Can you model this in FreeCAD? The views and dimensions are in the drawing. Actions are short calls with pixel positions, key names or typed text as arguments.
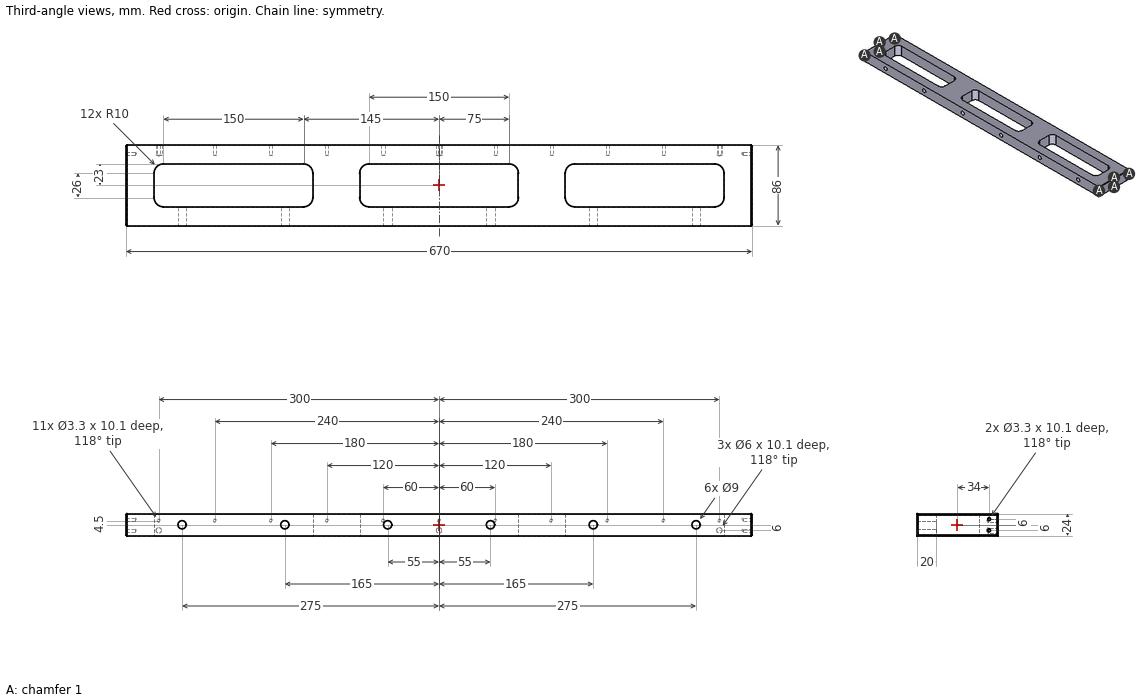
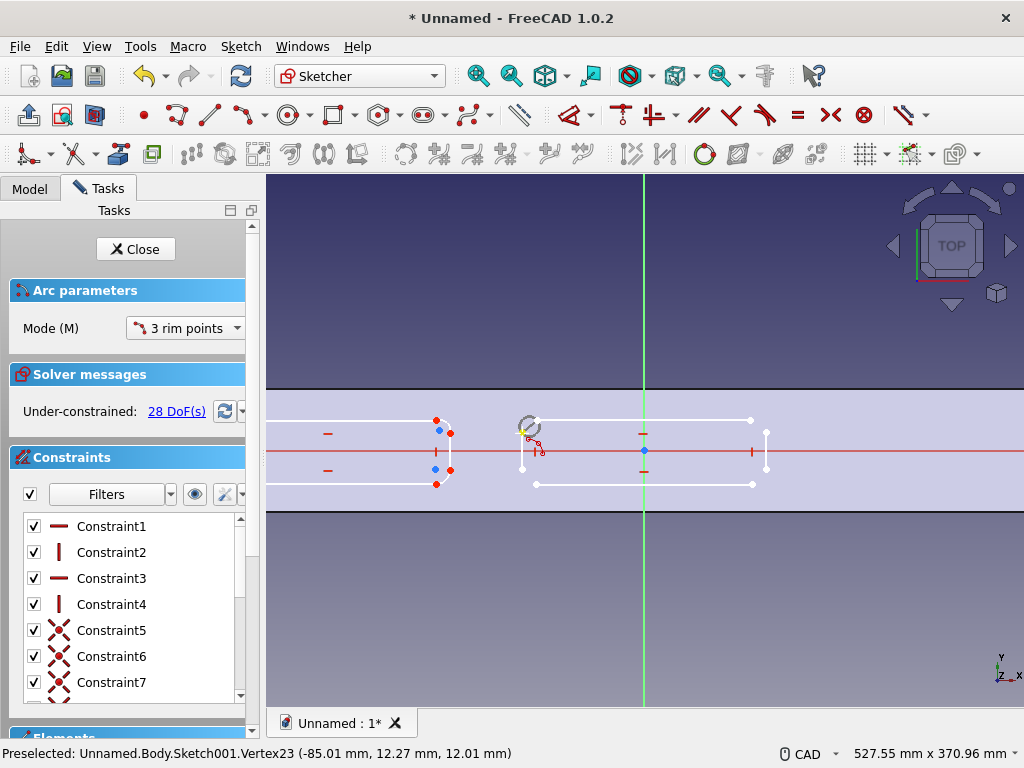
scroll(526, 422, up, 7)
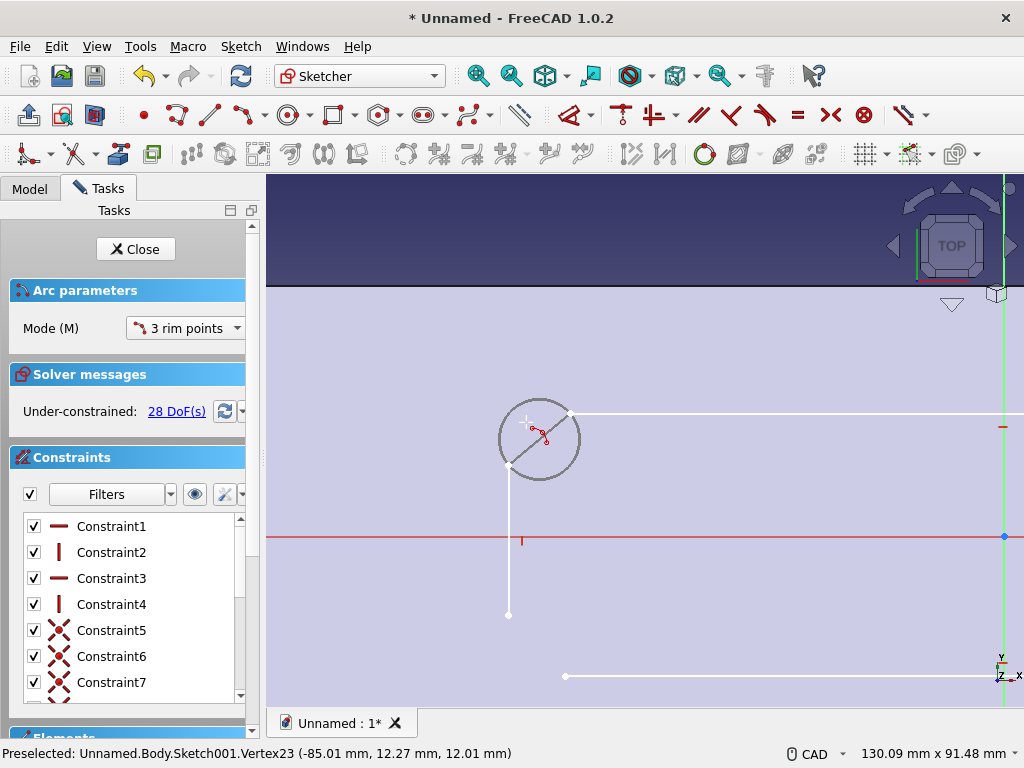
click(526, 420)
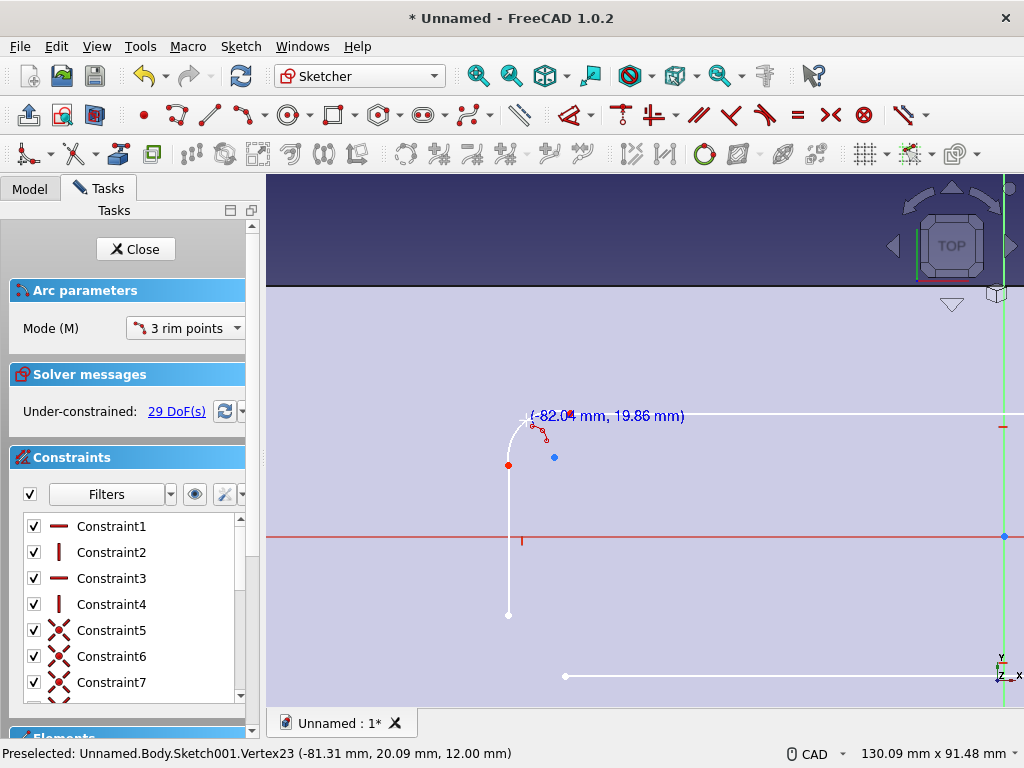
scroll(523, 429, down, 11)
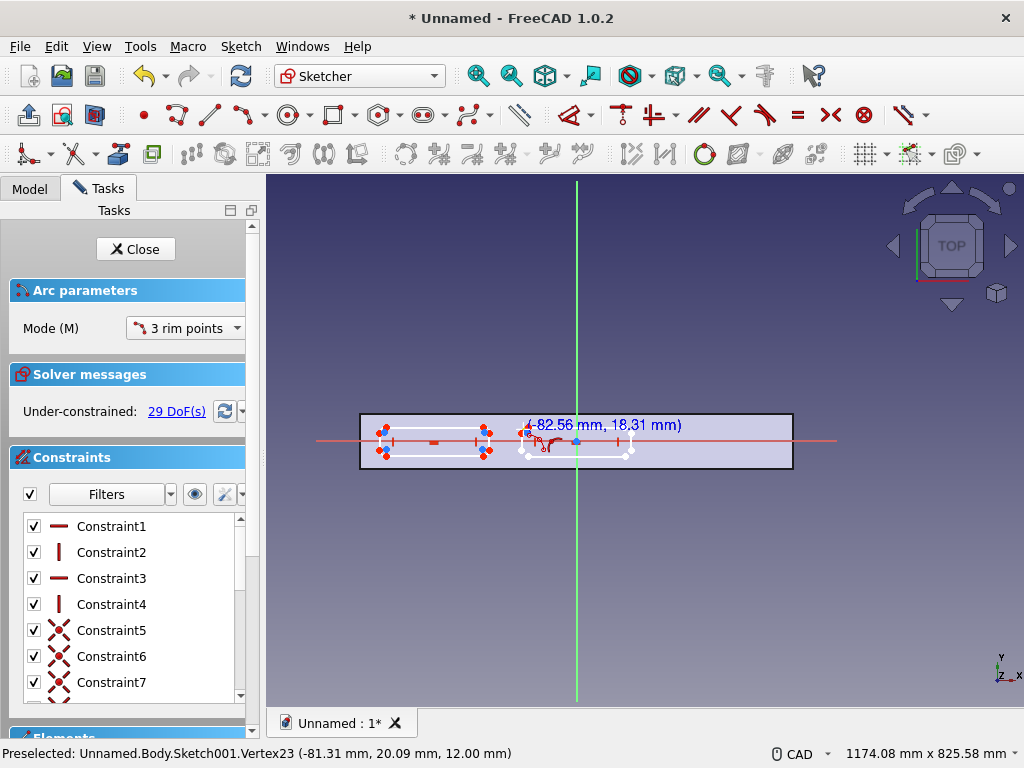
scroll(522, 450, up, 4)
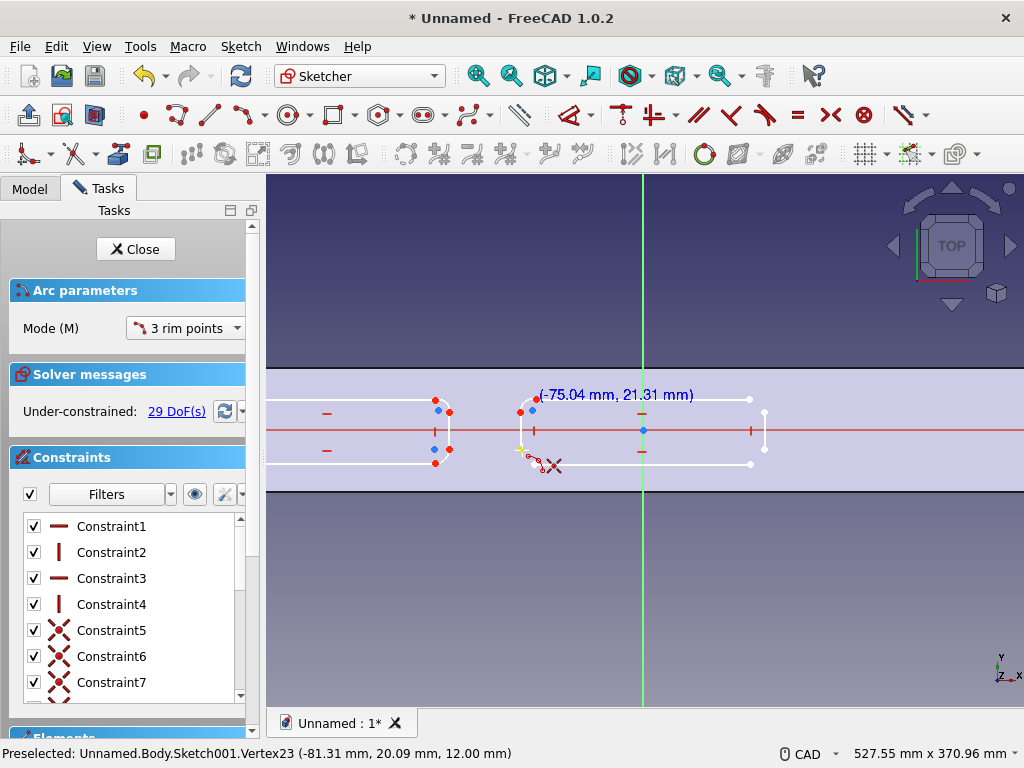
click(521, 449)
click(535, 464)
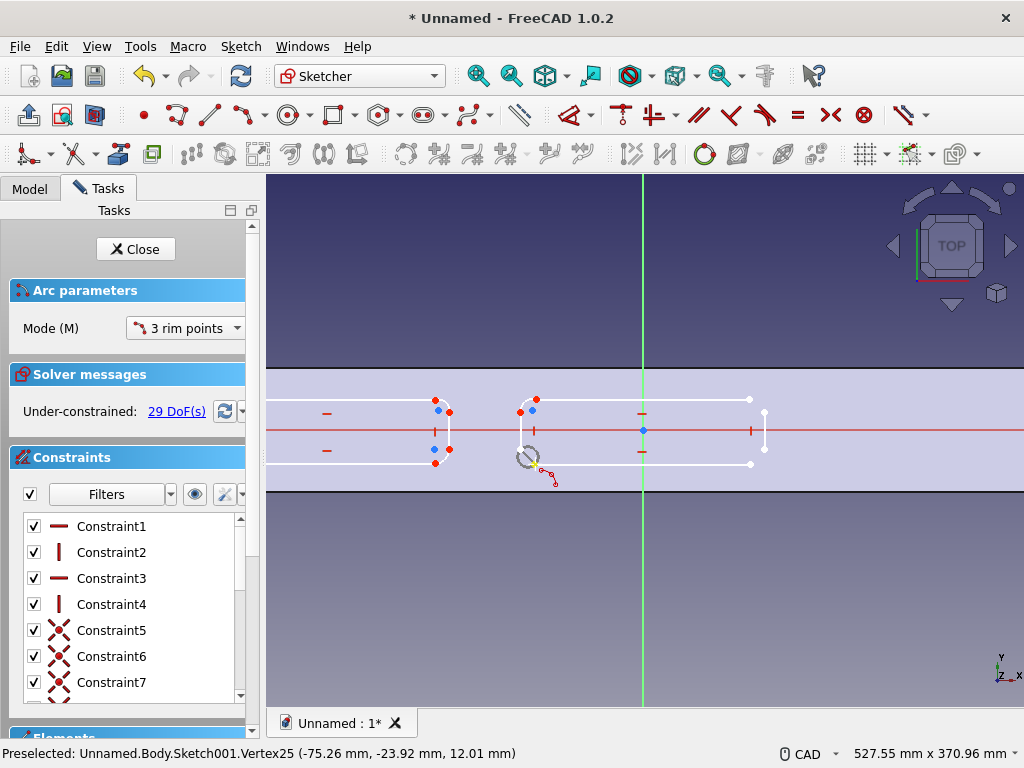
scroll(525, 459, up, 7)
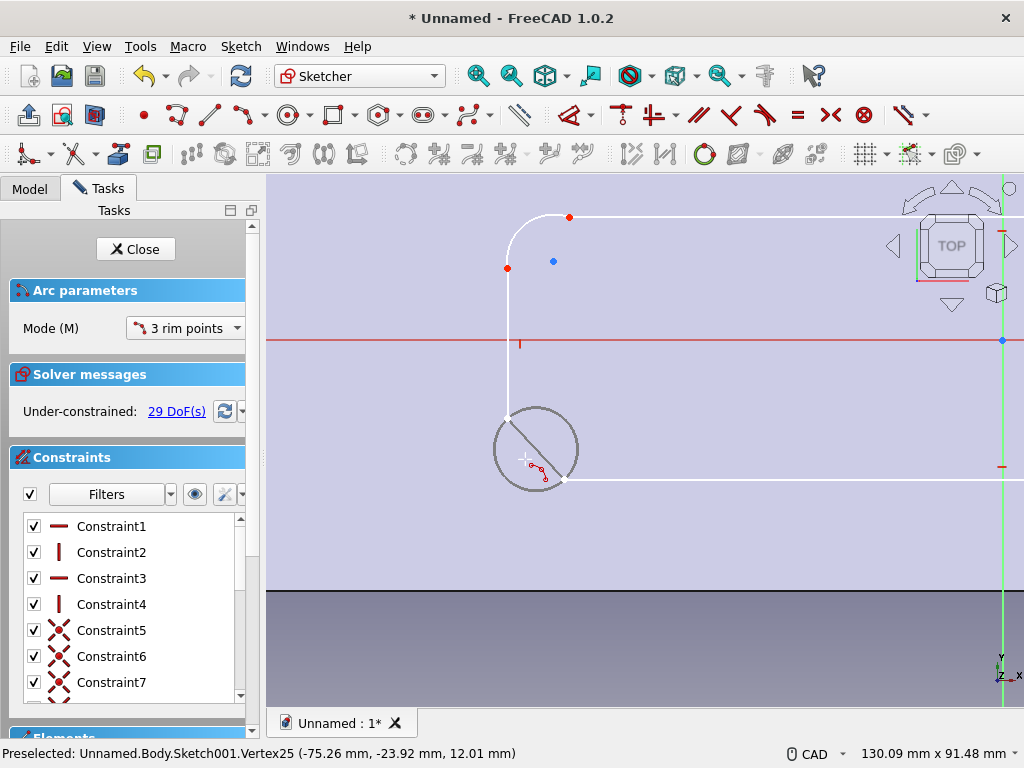
click(525, 457)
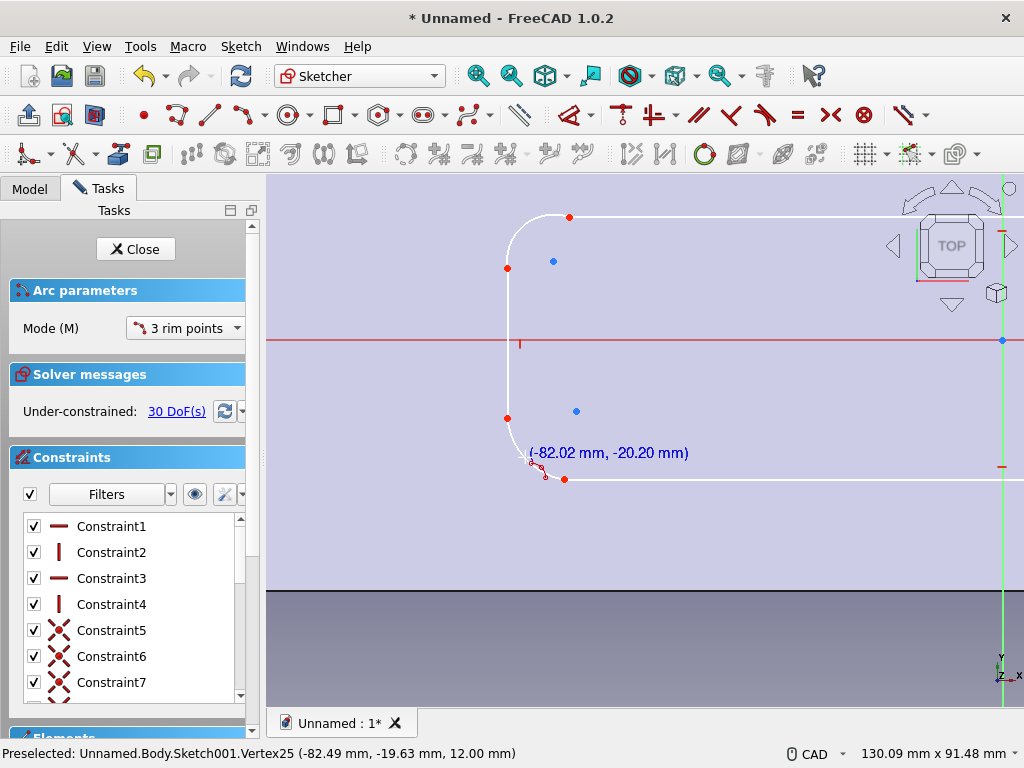
scroll(523, 453, down, 11)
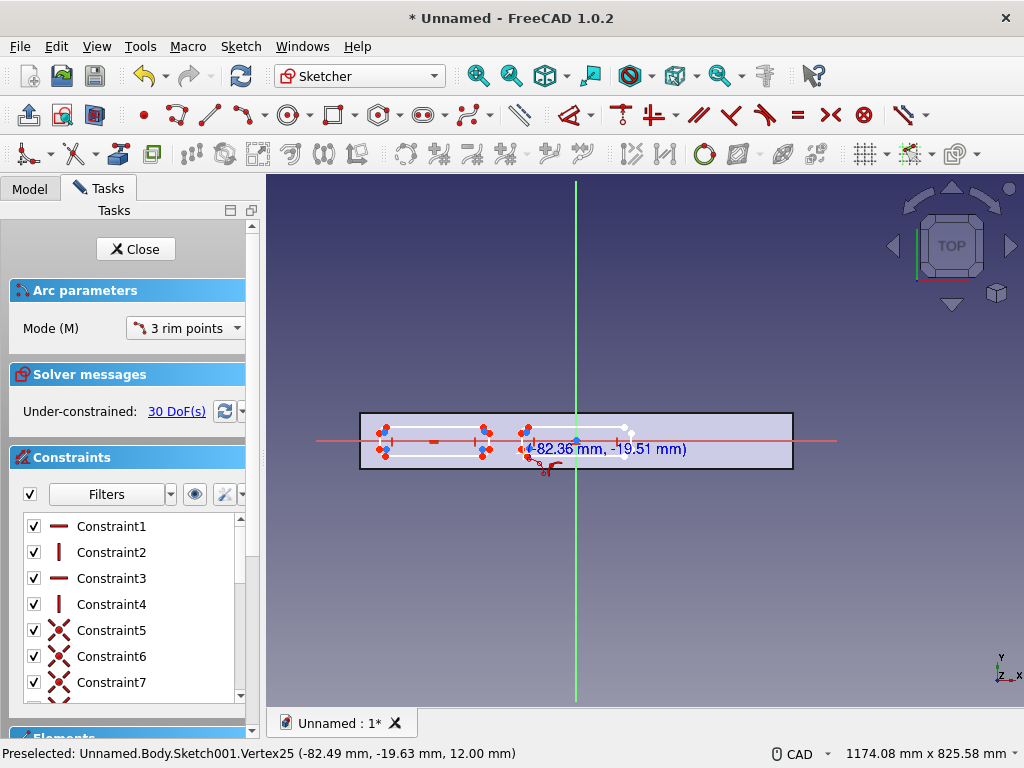
scroll(625, 456, up, 3)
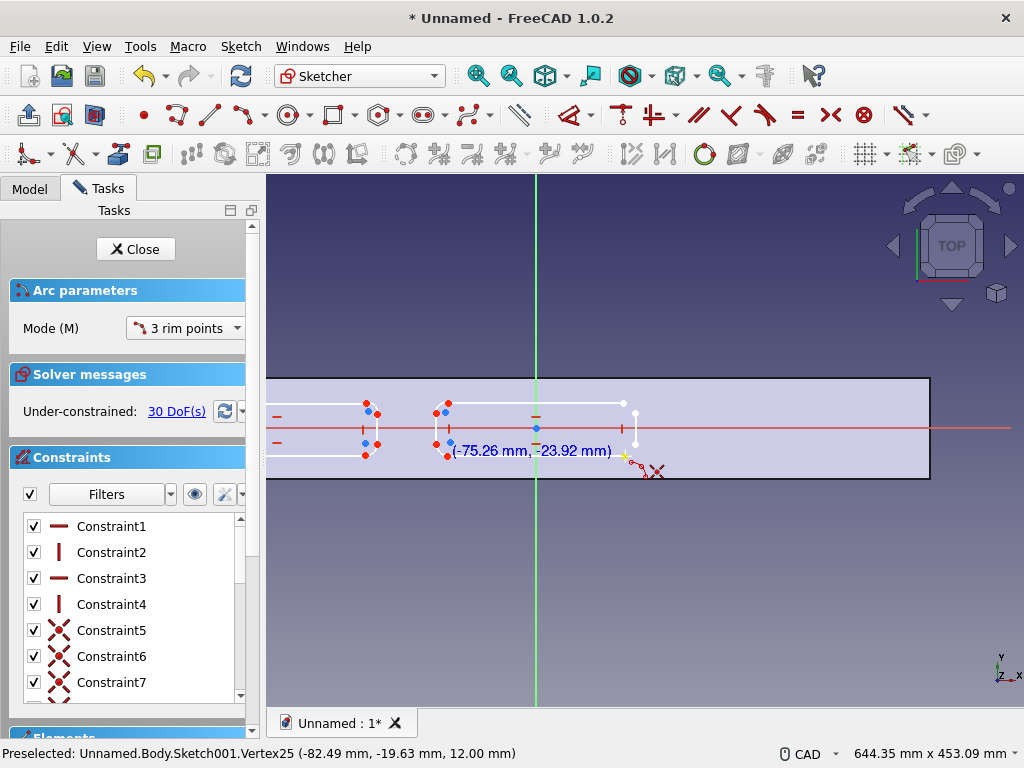
click(625, 456)
click(636, 444)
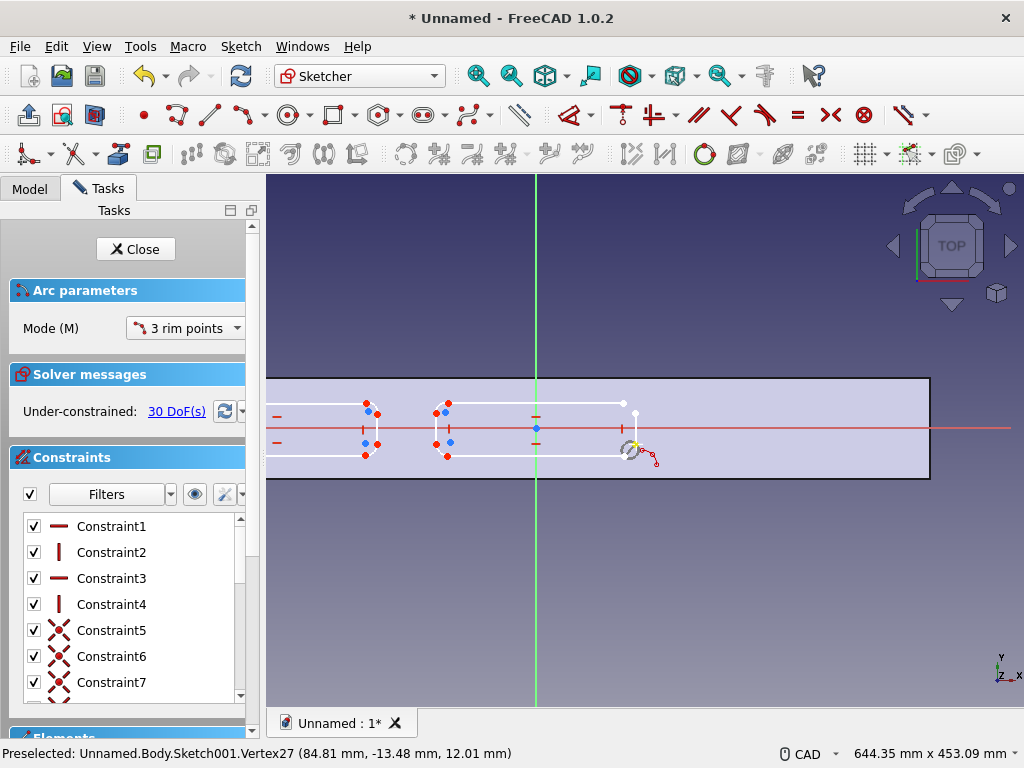
scroll(633, 452, up, 8)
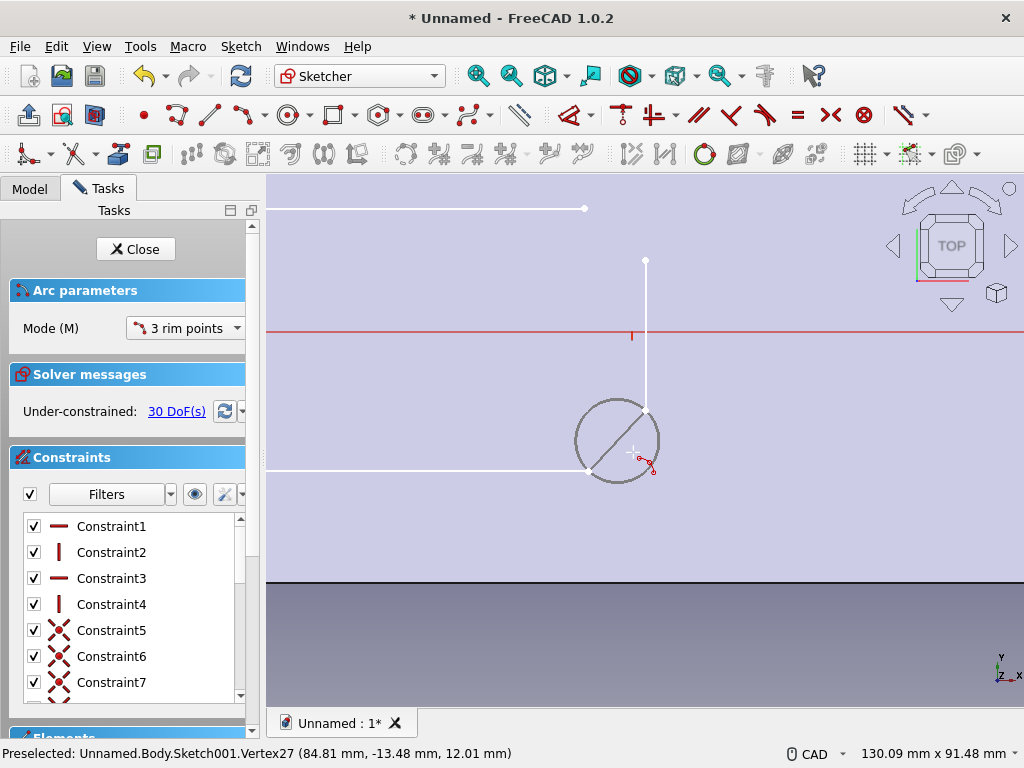
click(630, 449)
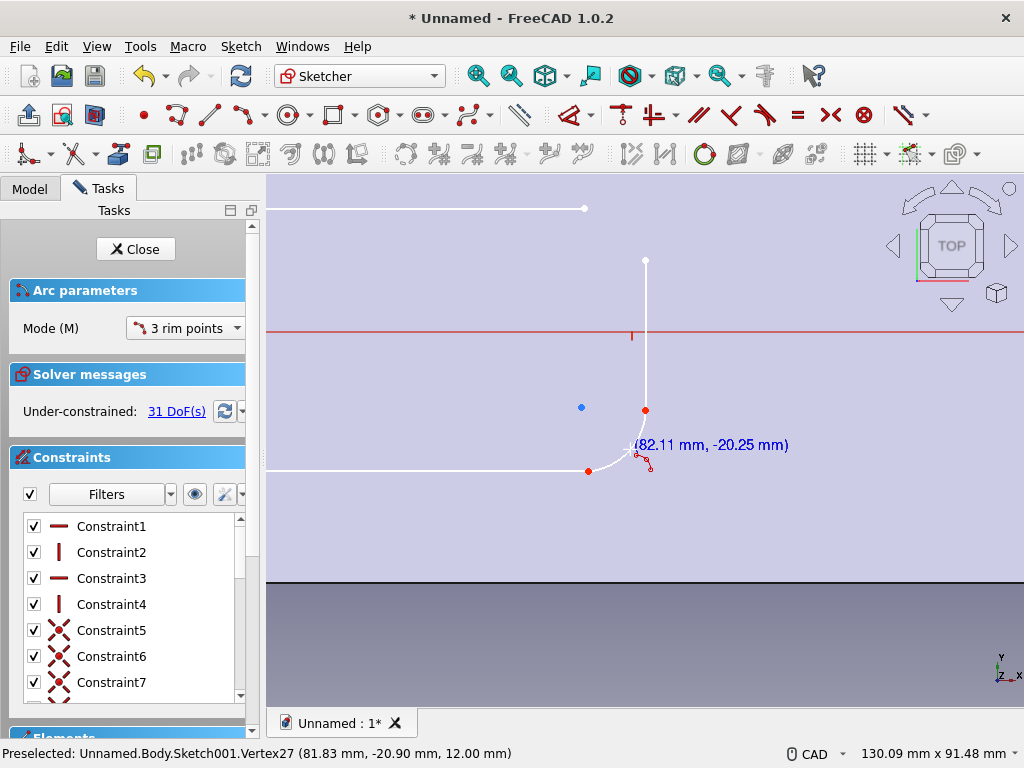
scroll(629, 454, down, 11)